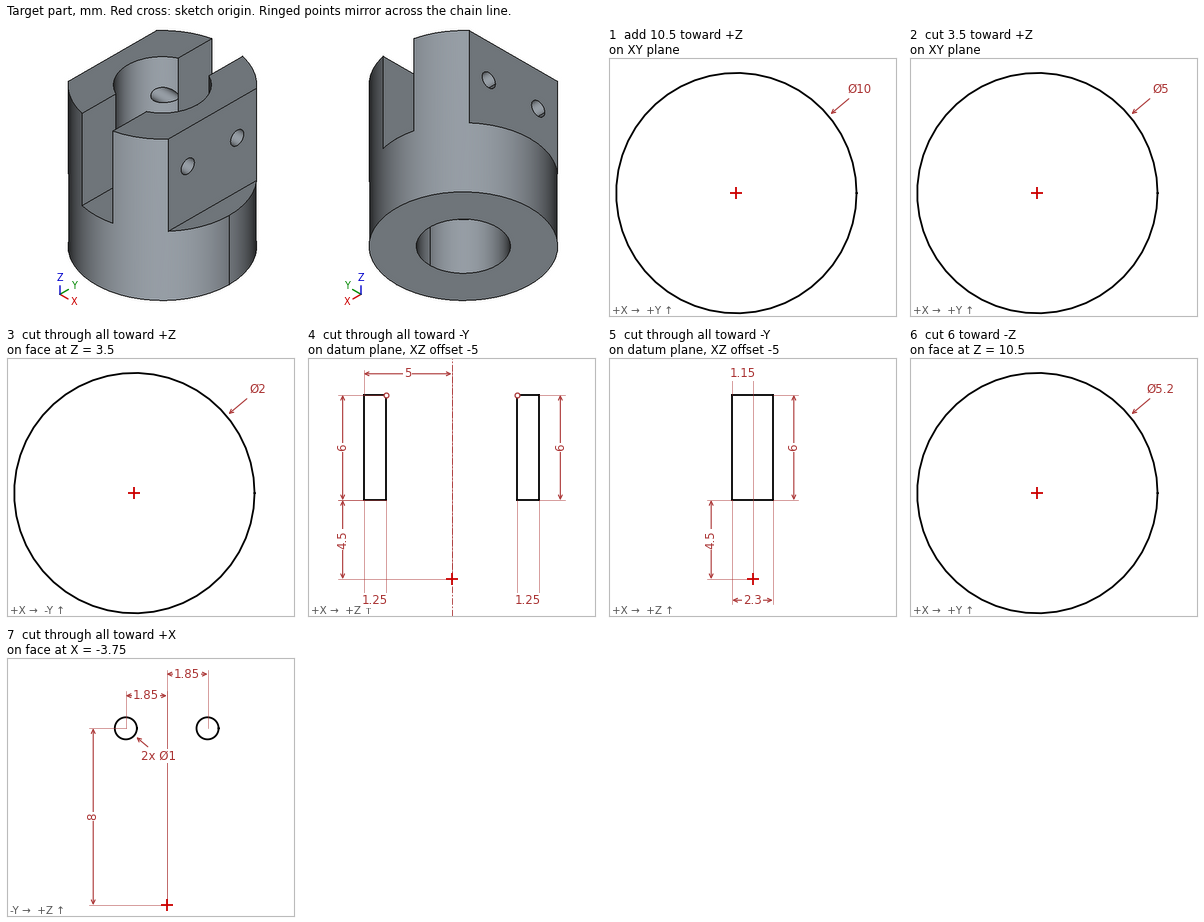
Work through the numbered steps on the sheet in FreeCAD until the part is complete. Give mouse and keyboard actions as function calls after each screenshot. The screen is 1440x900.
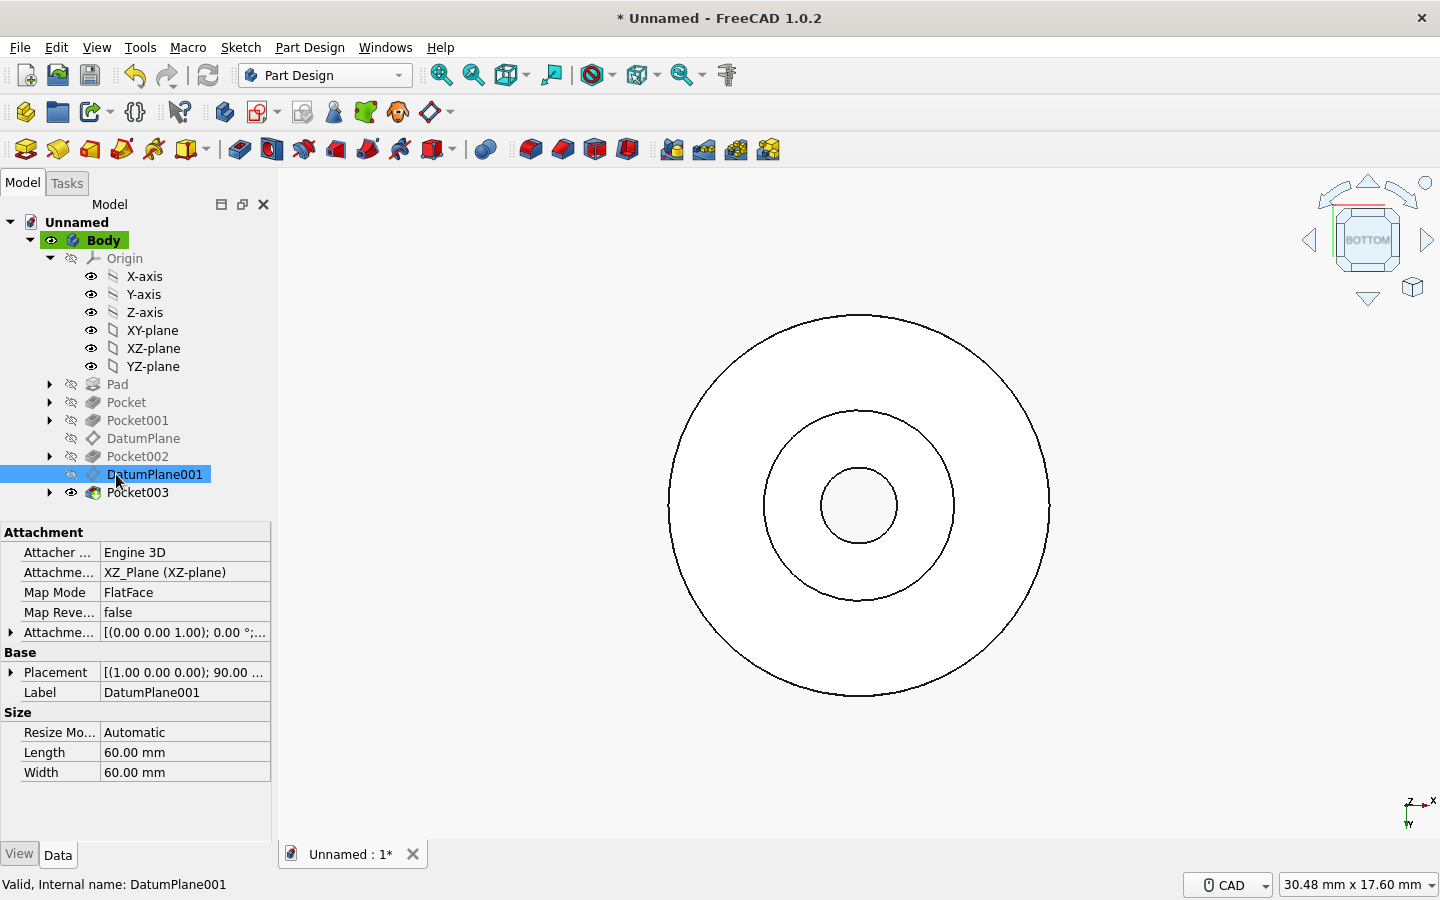
key(0)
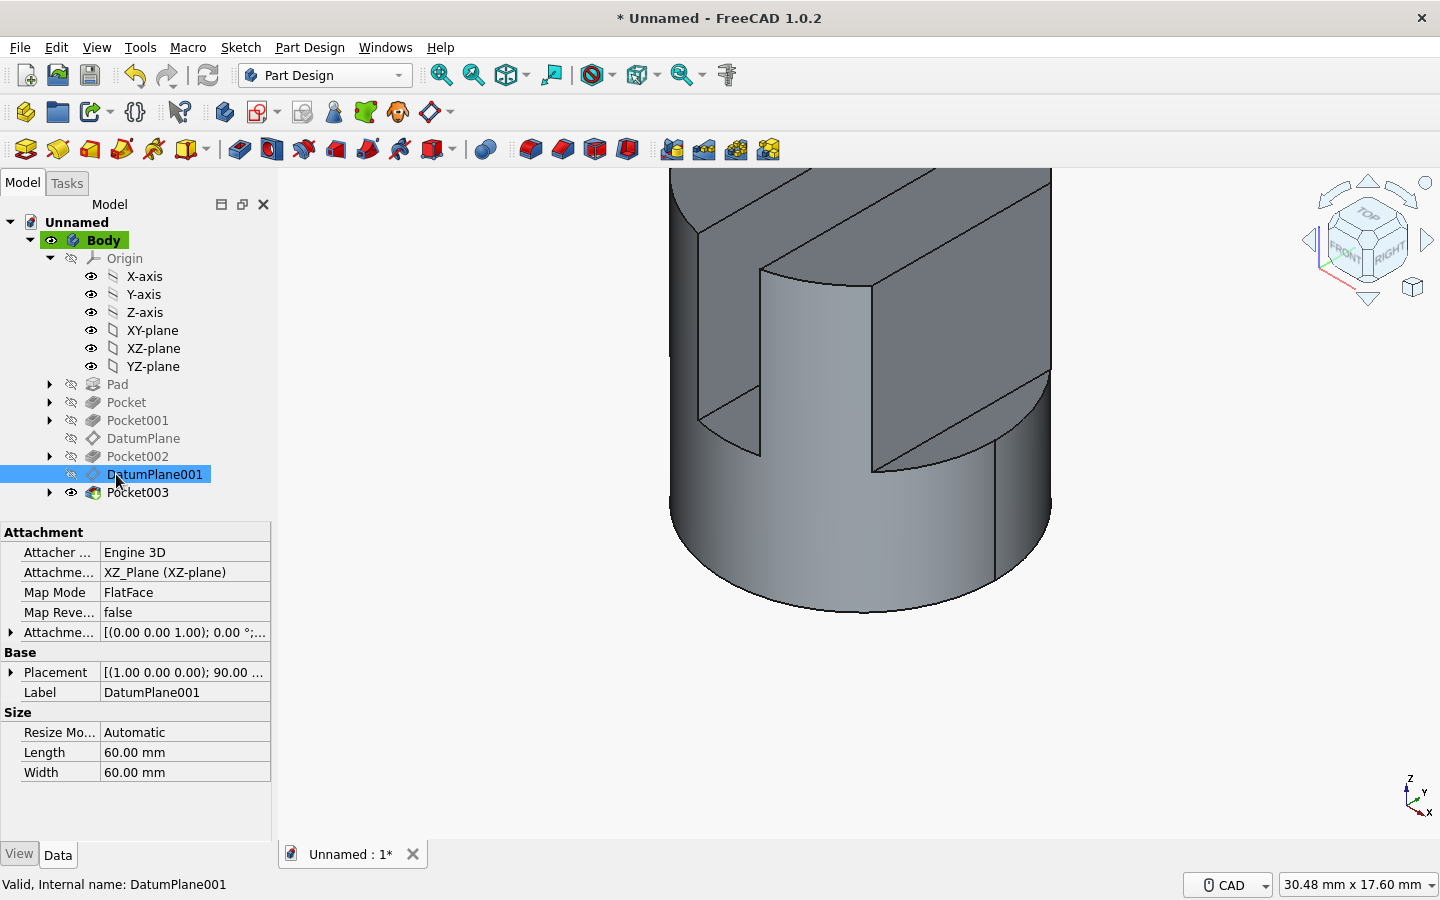
key(v)
key(f)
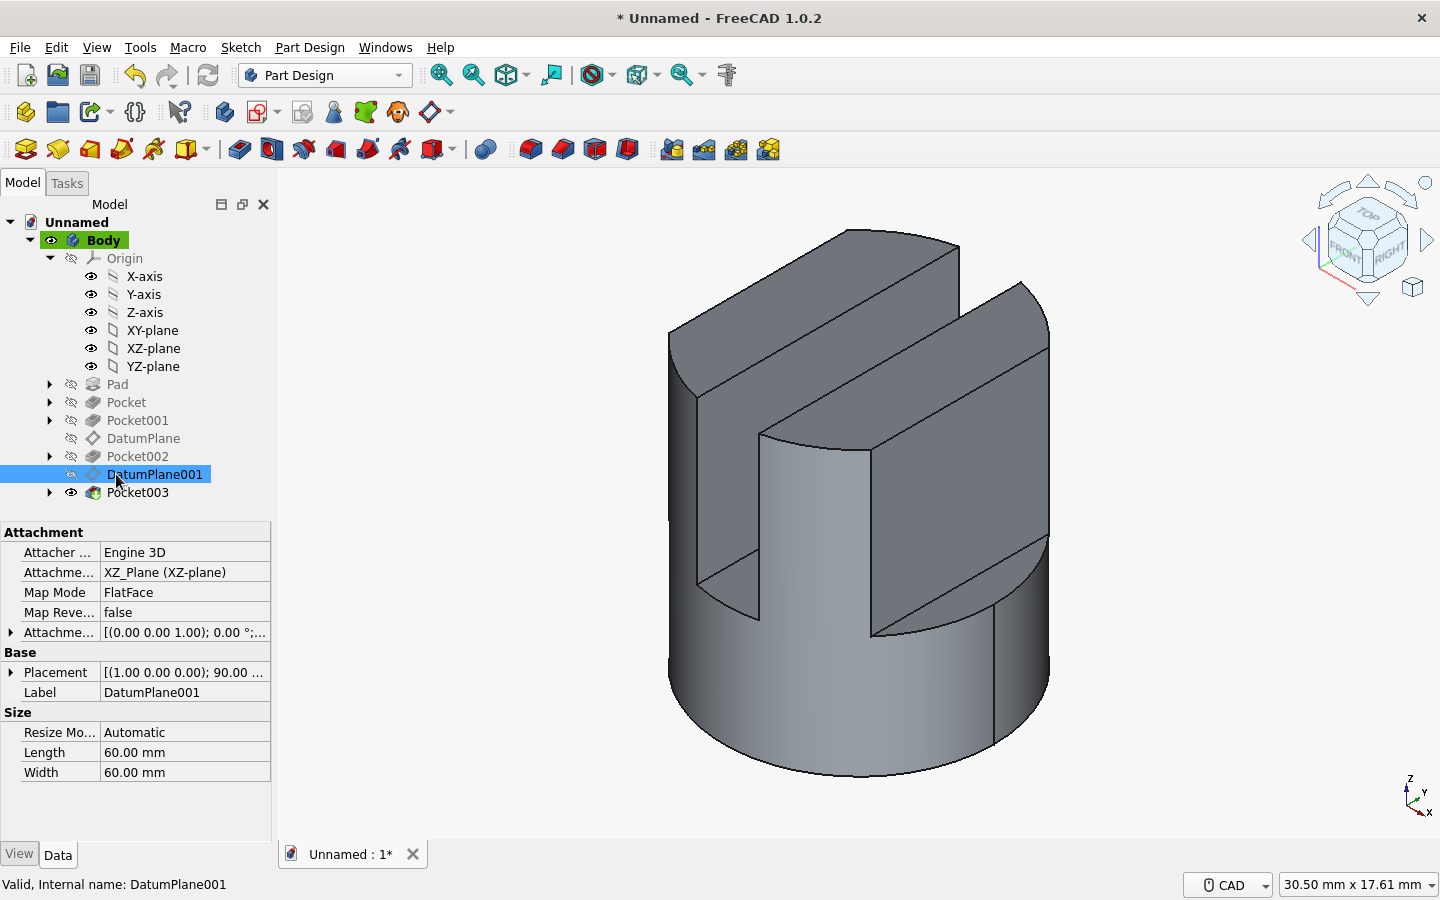
click(962, 356)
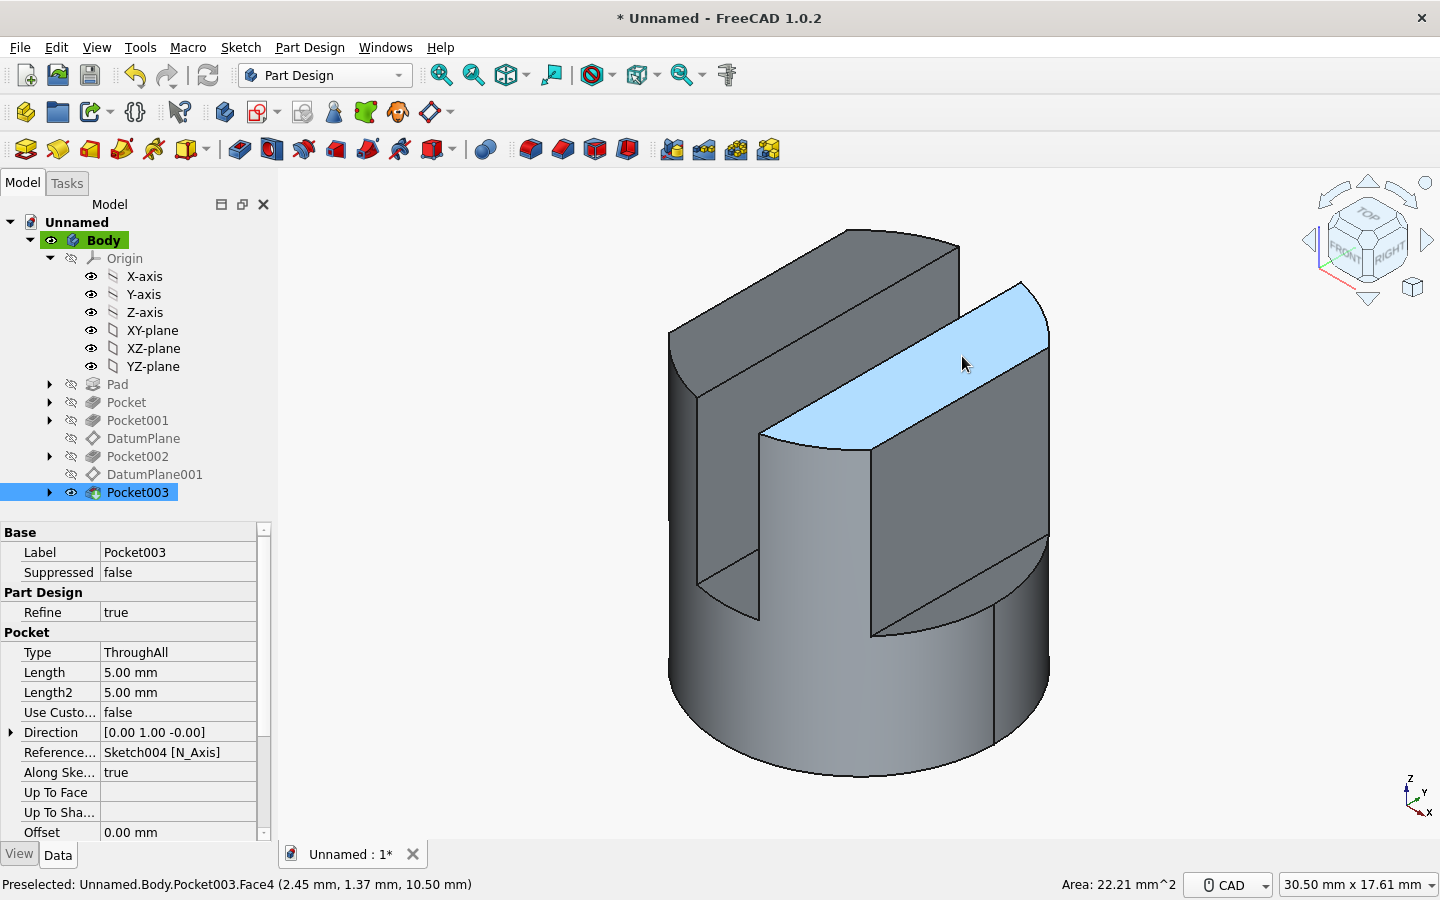
click(258, 112)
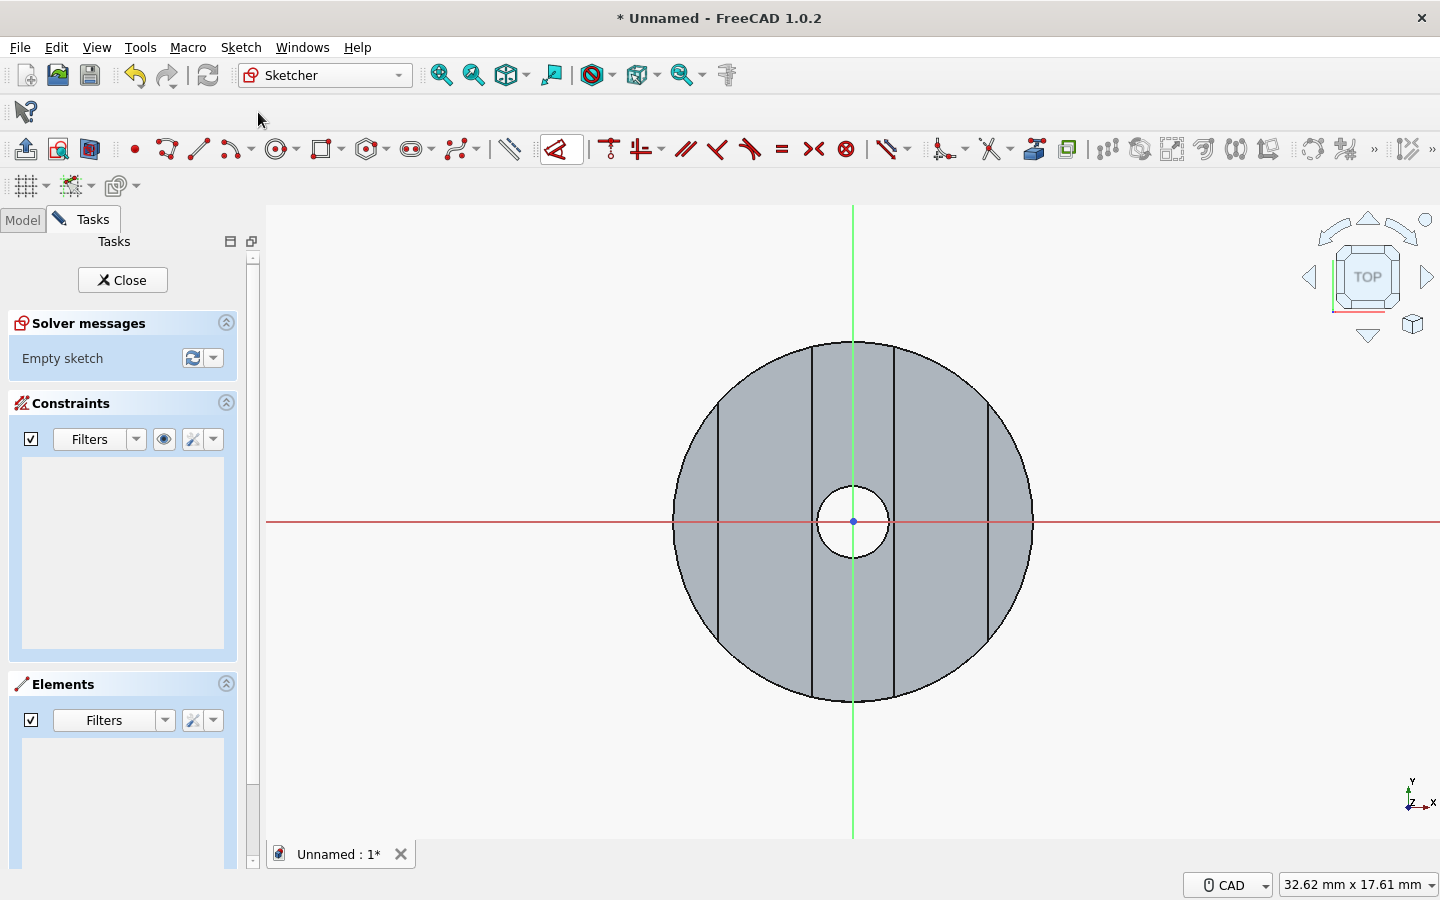
scroll(909, 522, up, 4)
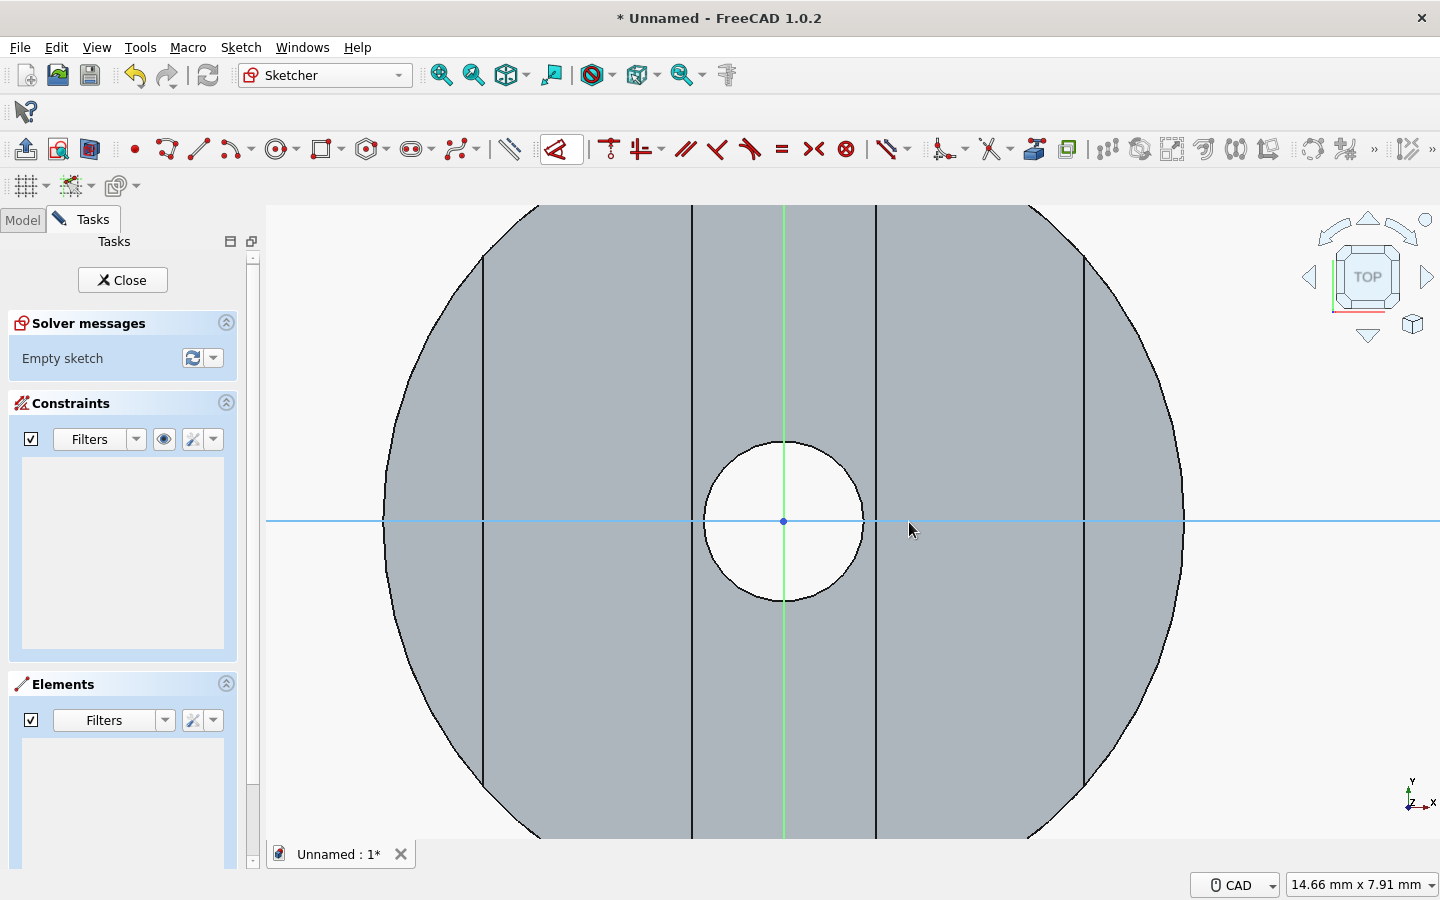
click(276, 150)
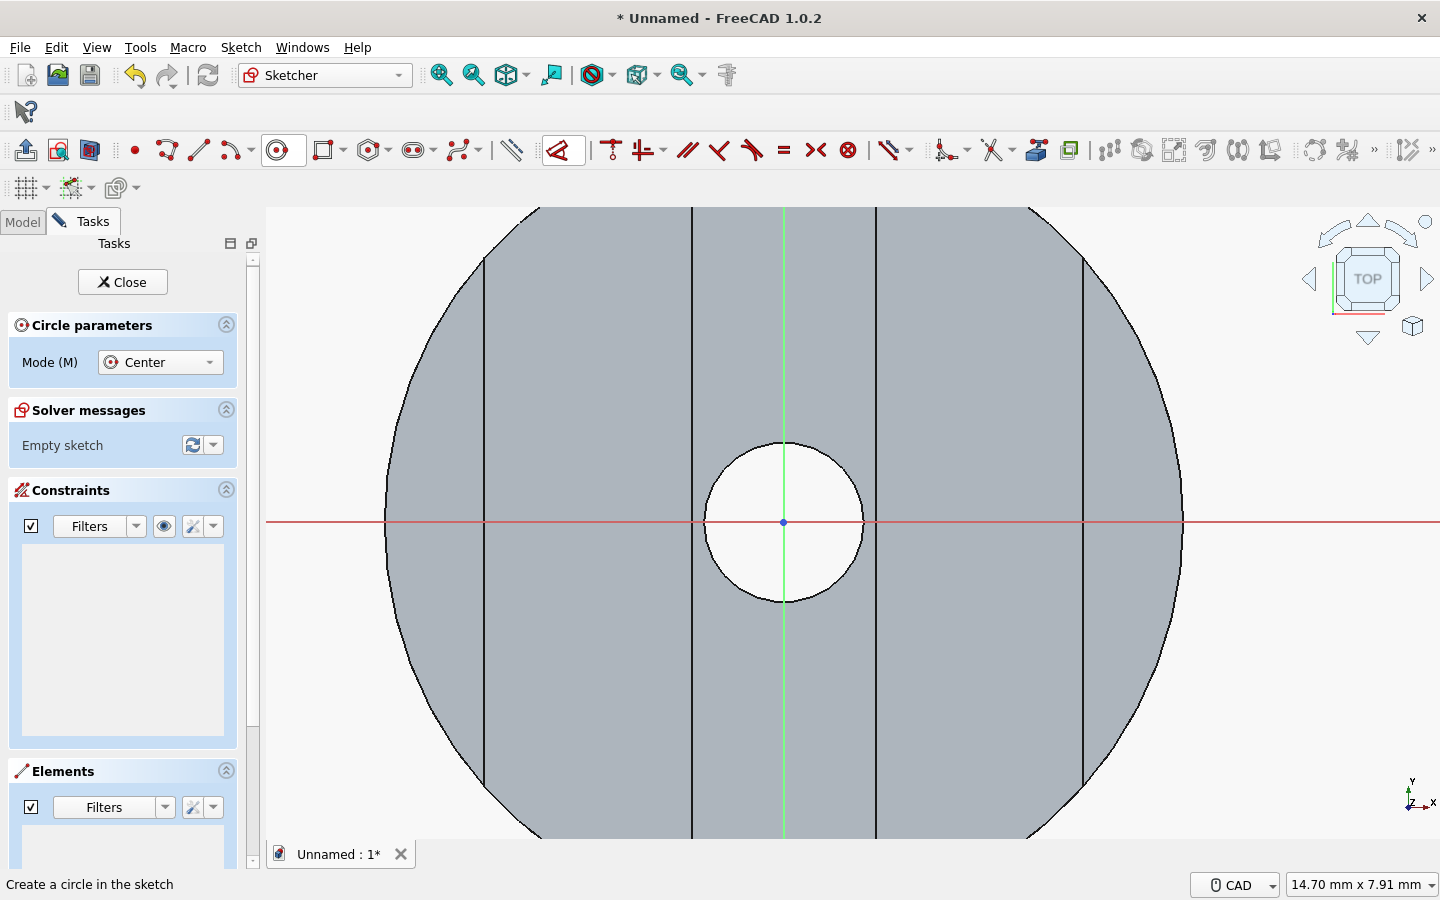
click(784, 522)
move(931, 376)